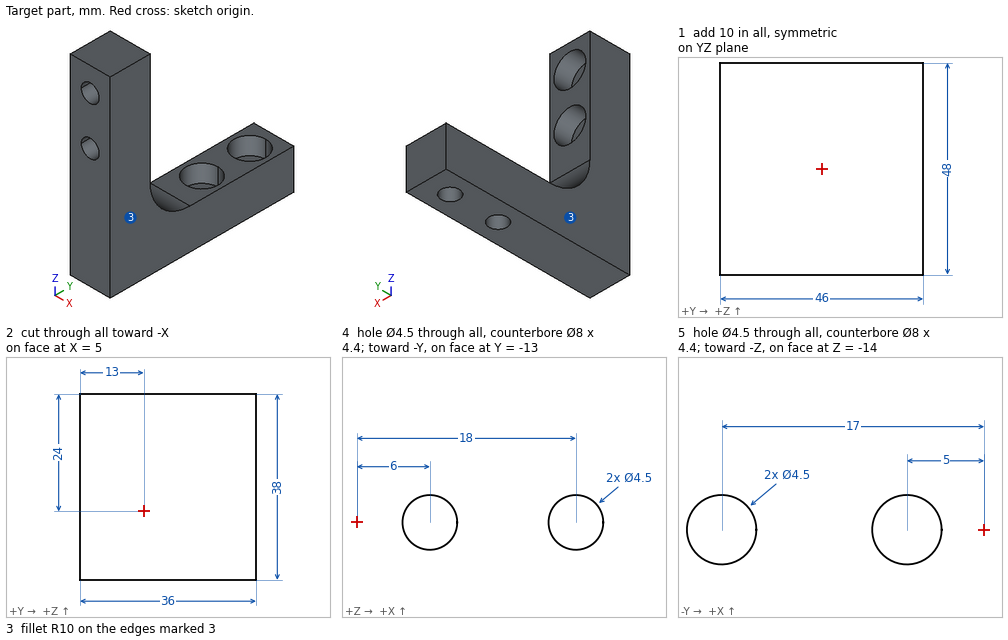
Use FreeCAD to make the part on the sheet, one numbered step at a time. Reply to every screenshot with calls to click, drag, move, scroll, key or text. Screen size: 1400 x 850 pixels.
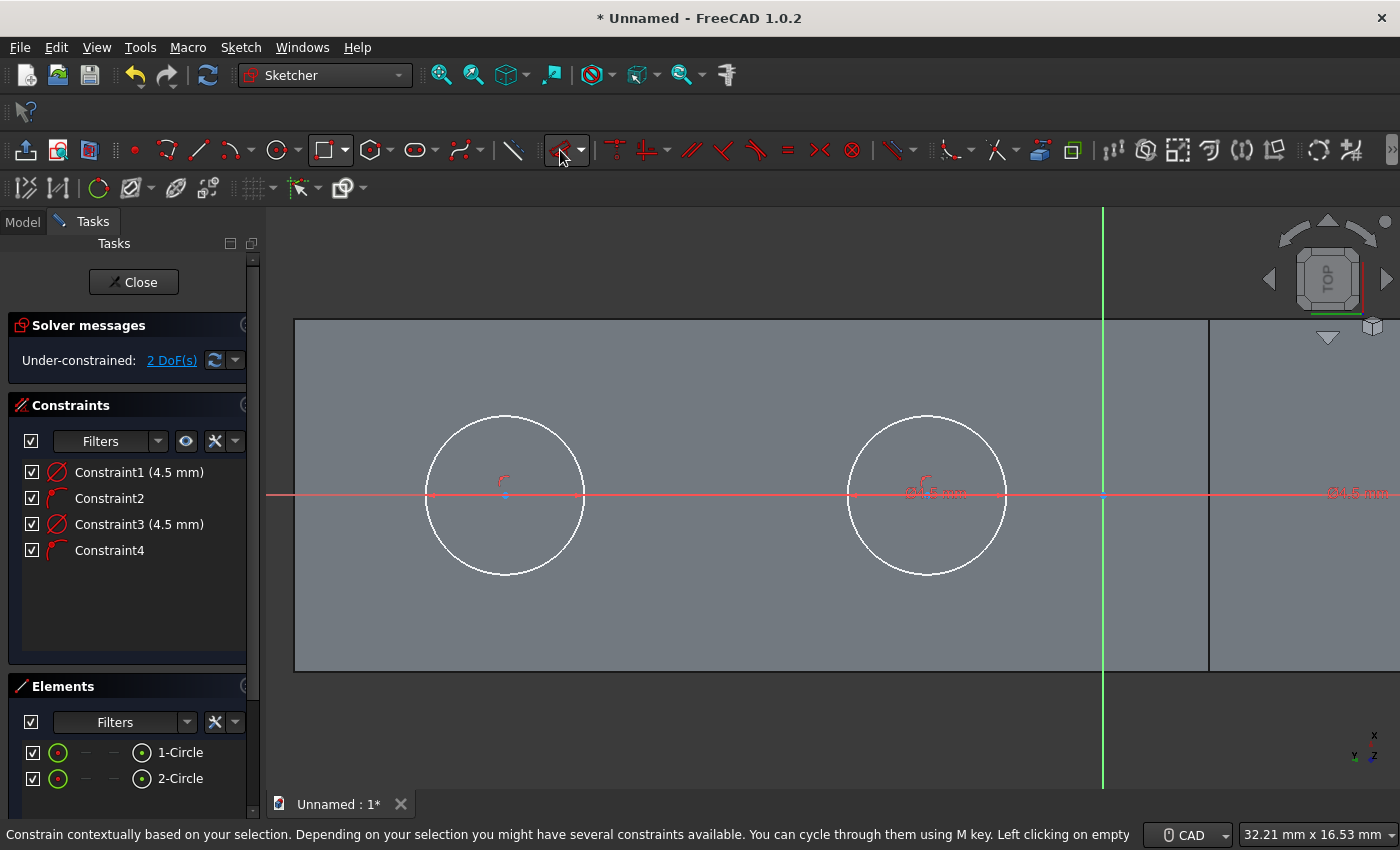
click(927, 495)
click(1015, 461)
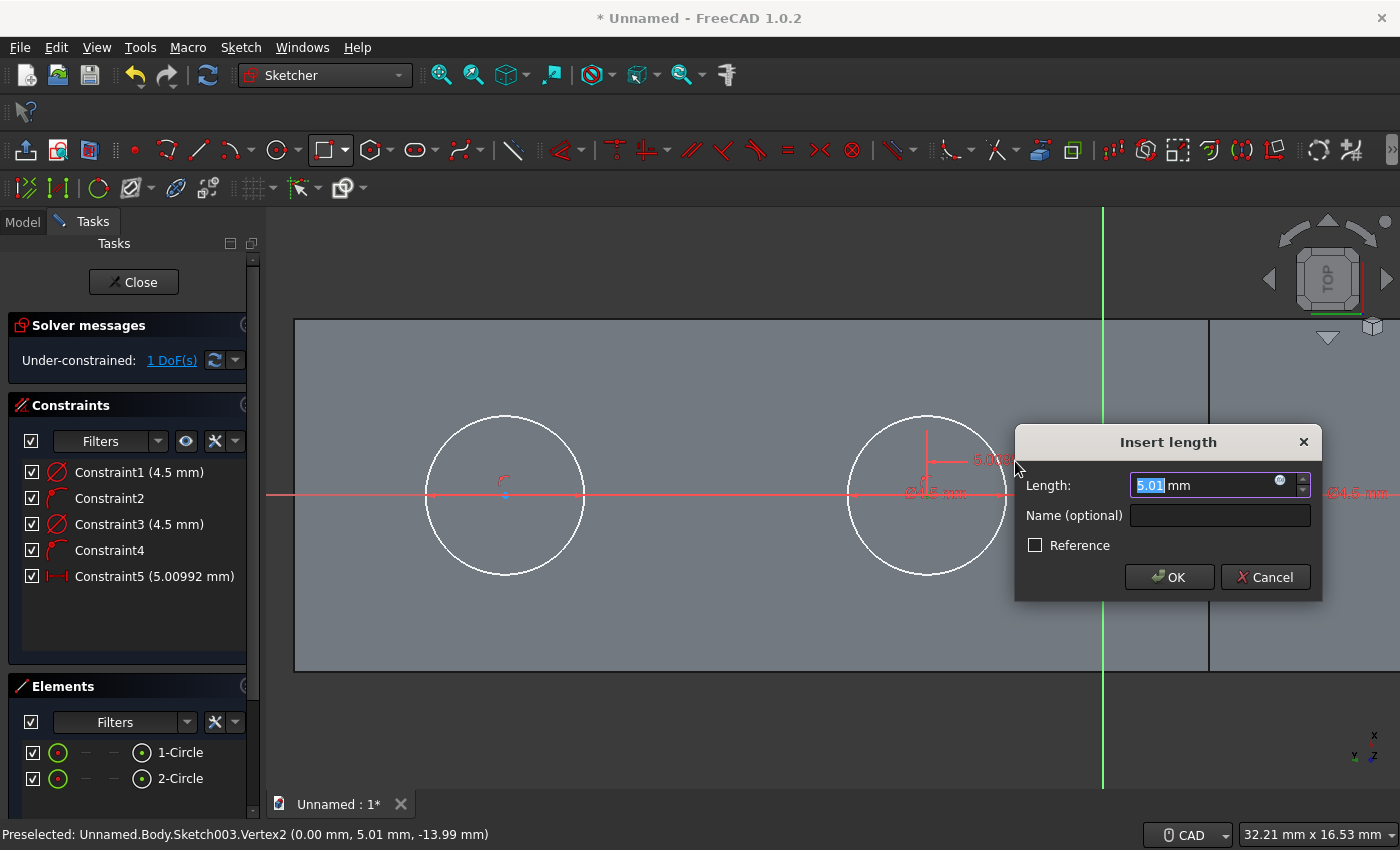
text(5)
key(Return)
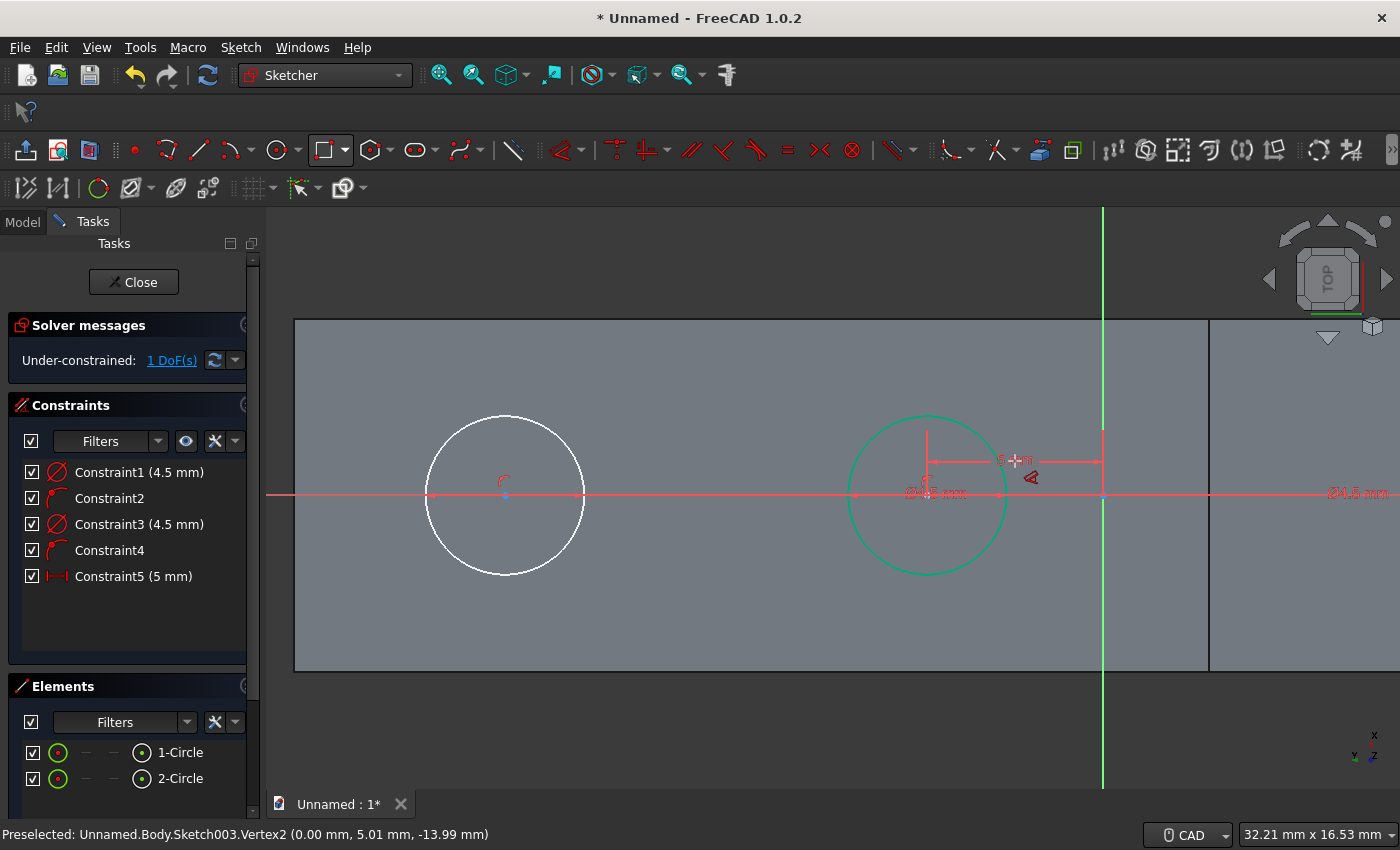
click(505, 495)
click(804, 529)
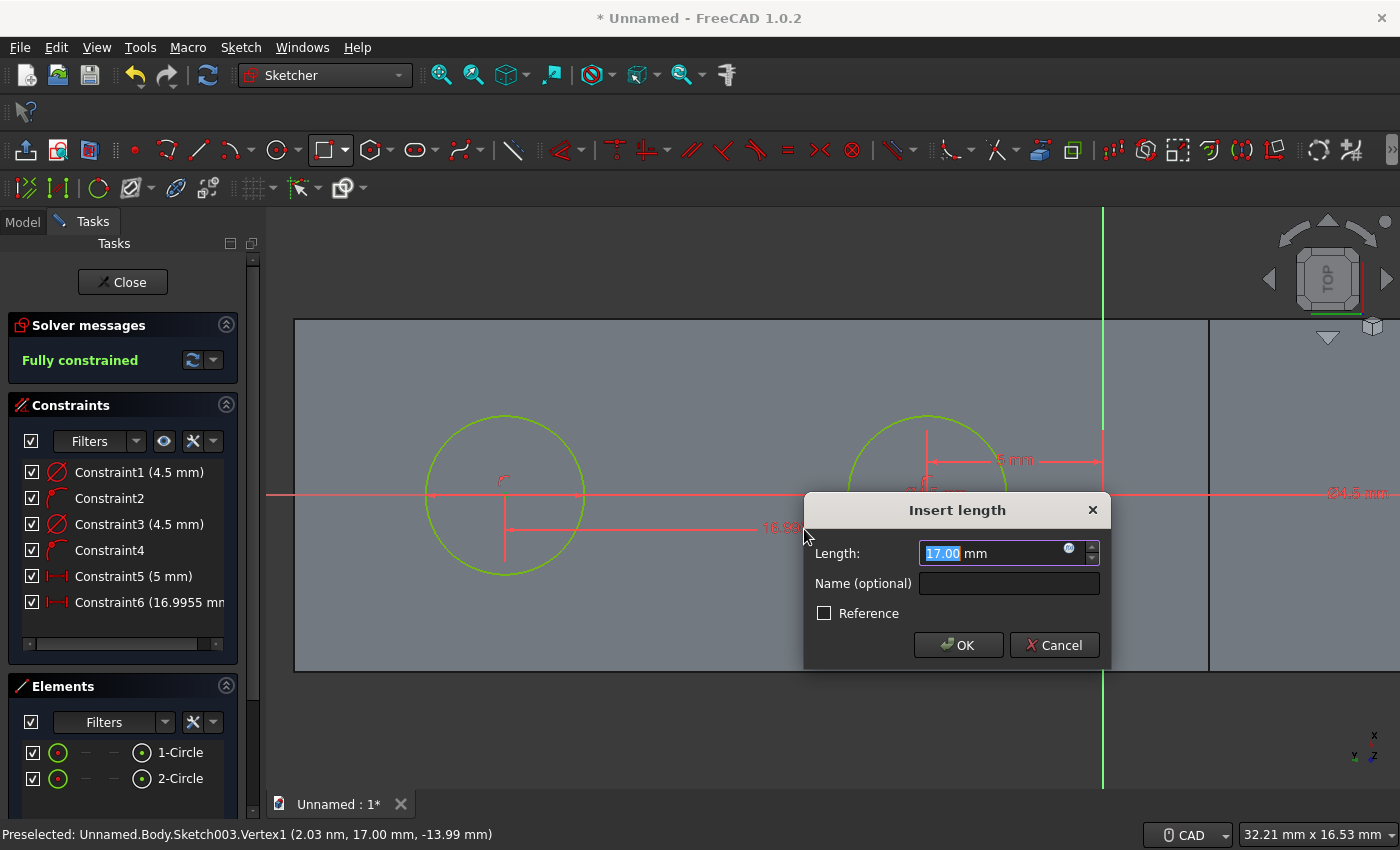
text(17)
key(Return)
key(Escape)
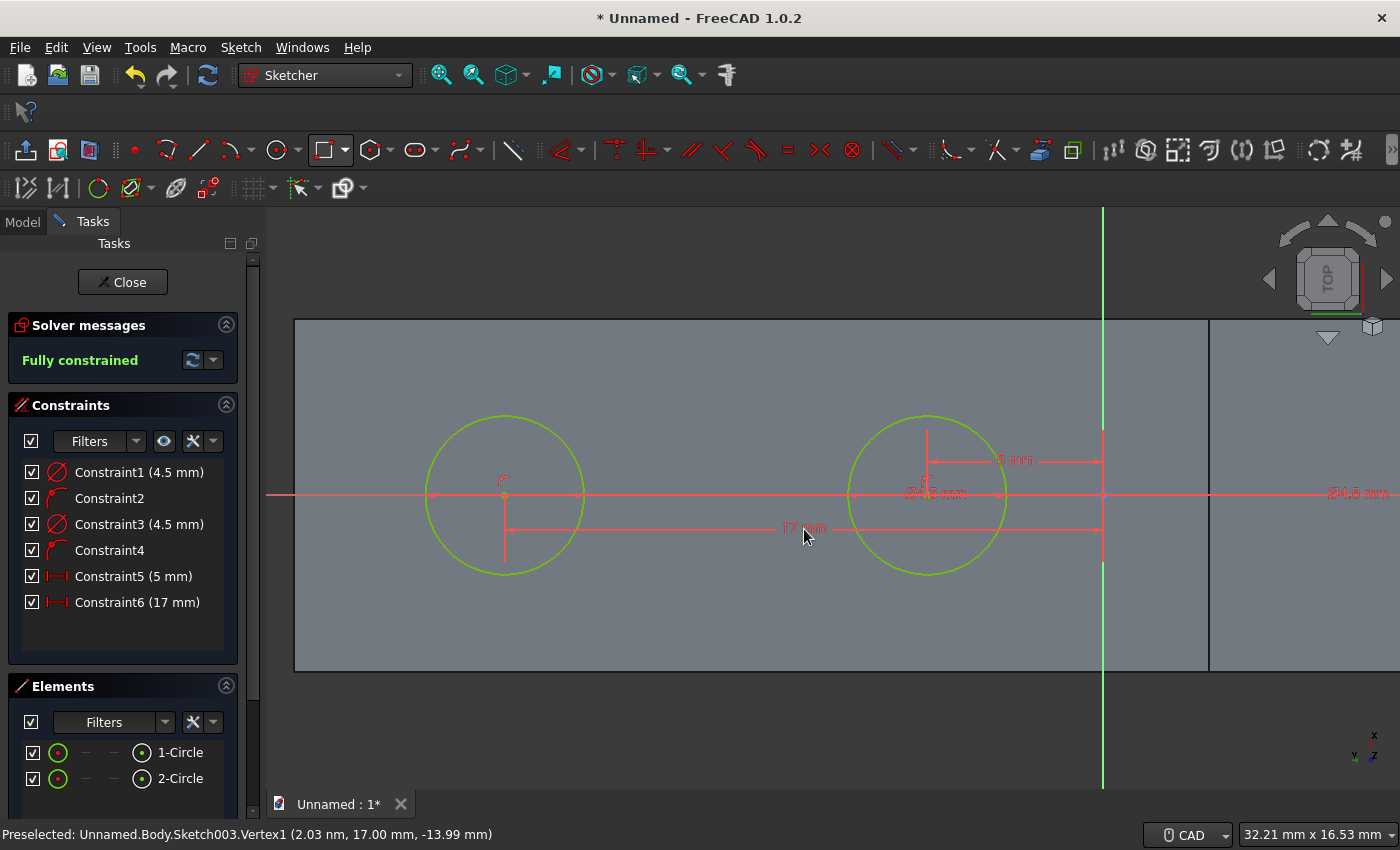
click(123, 282)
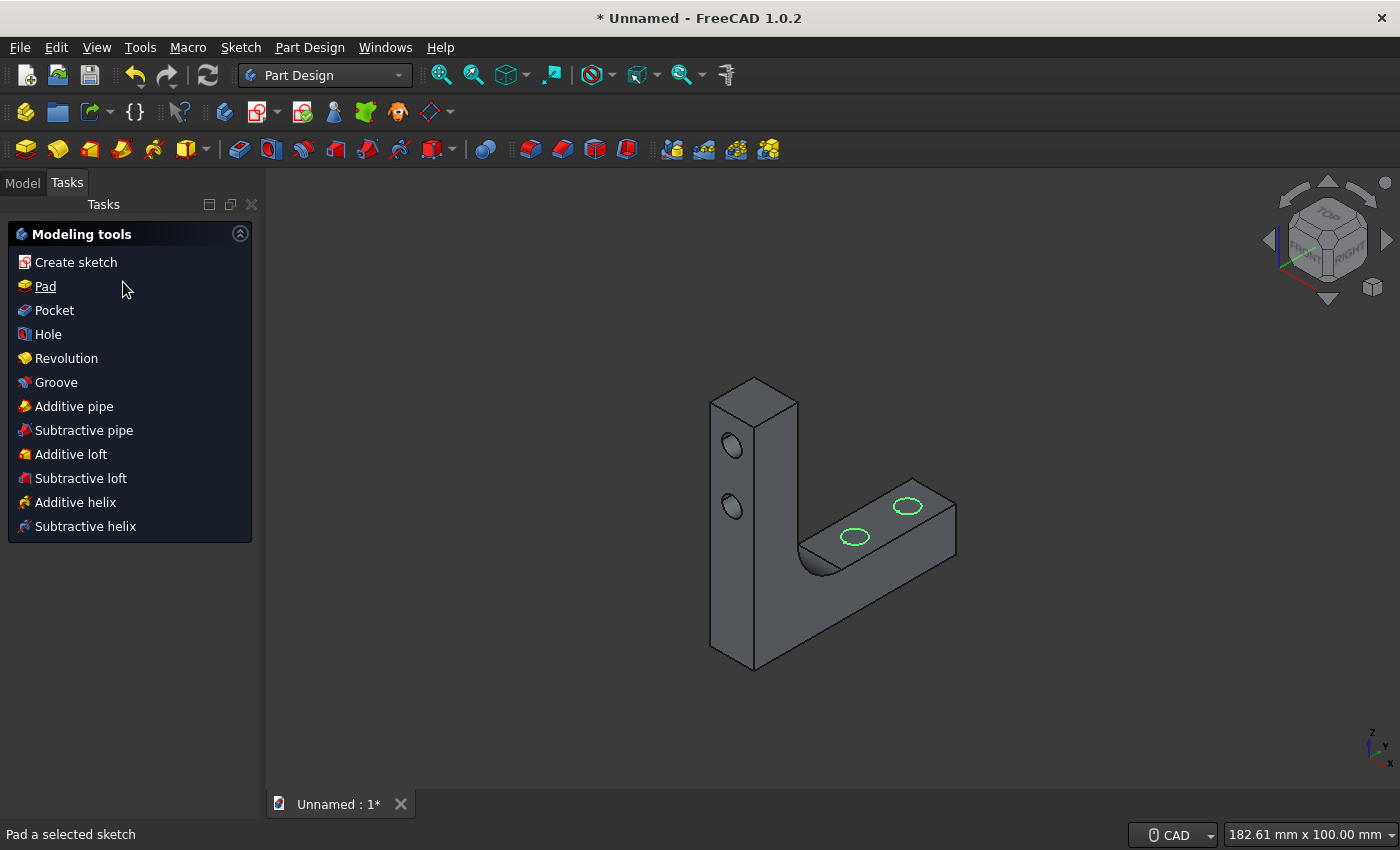
click(272, 150)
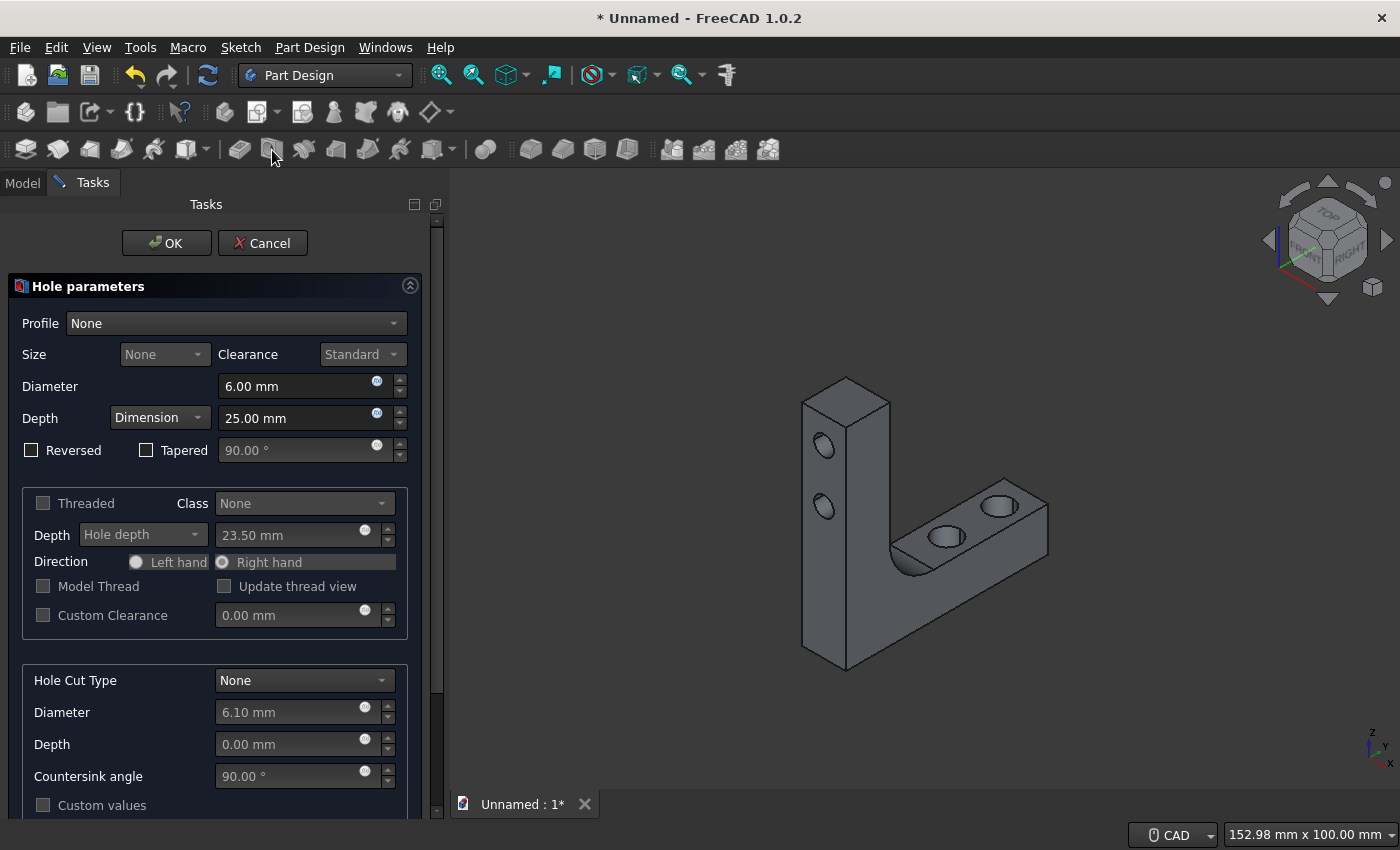
triple_click(305, 386)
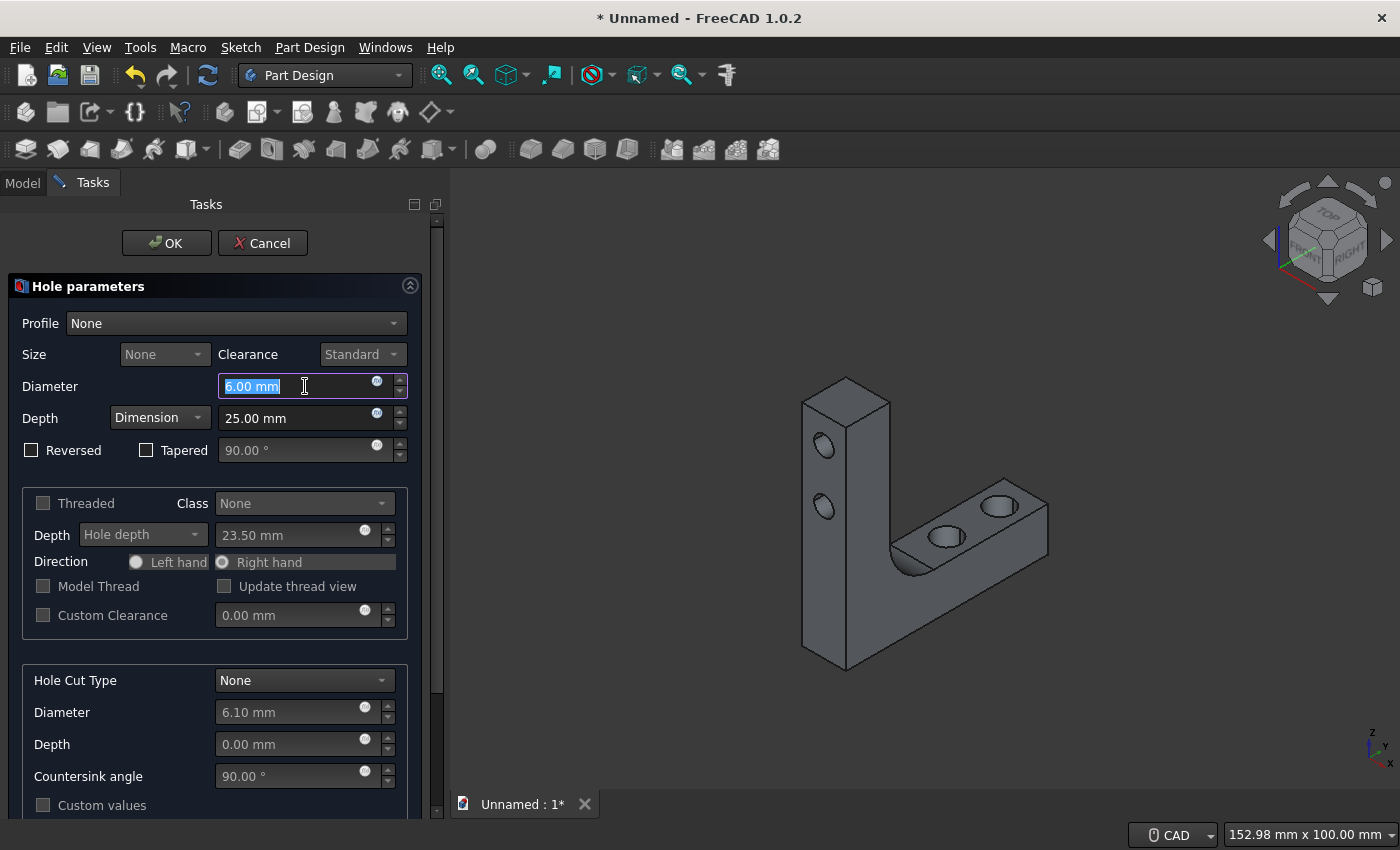
text(4.5)
key(Tab)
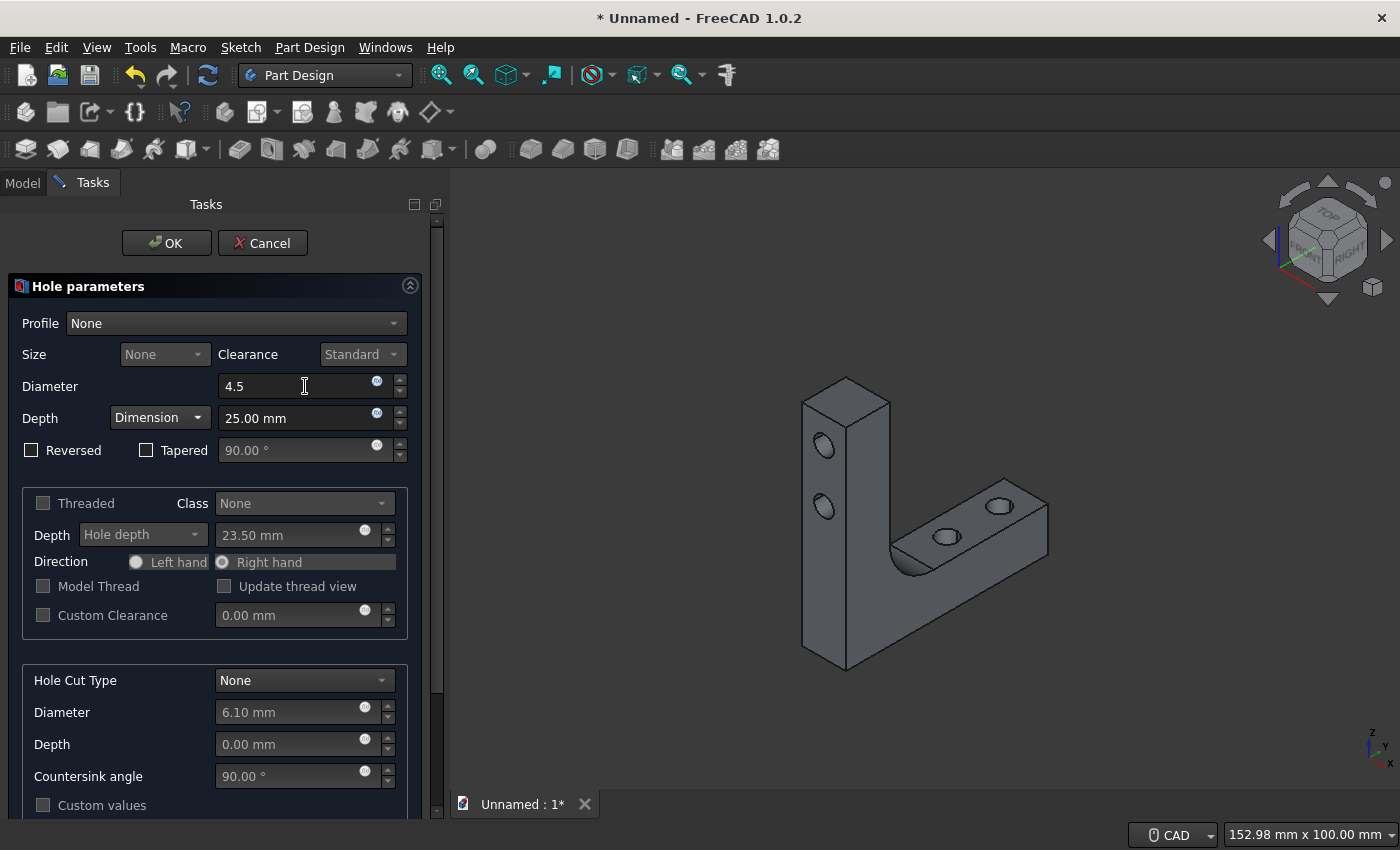
click(161, 418)